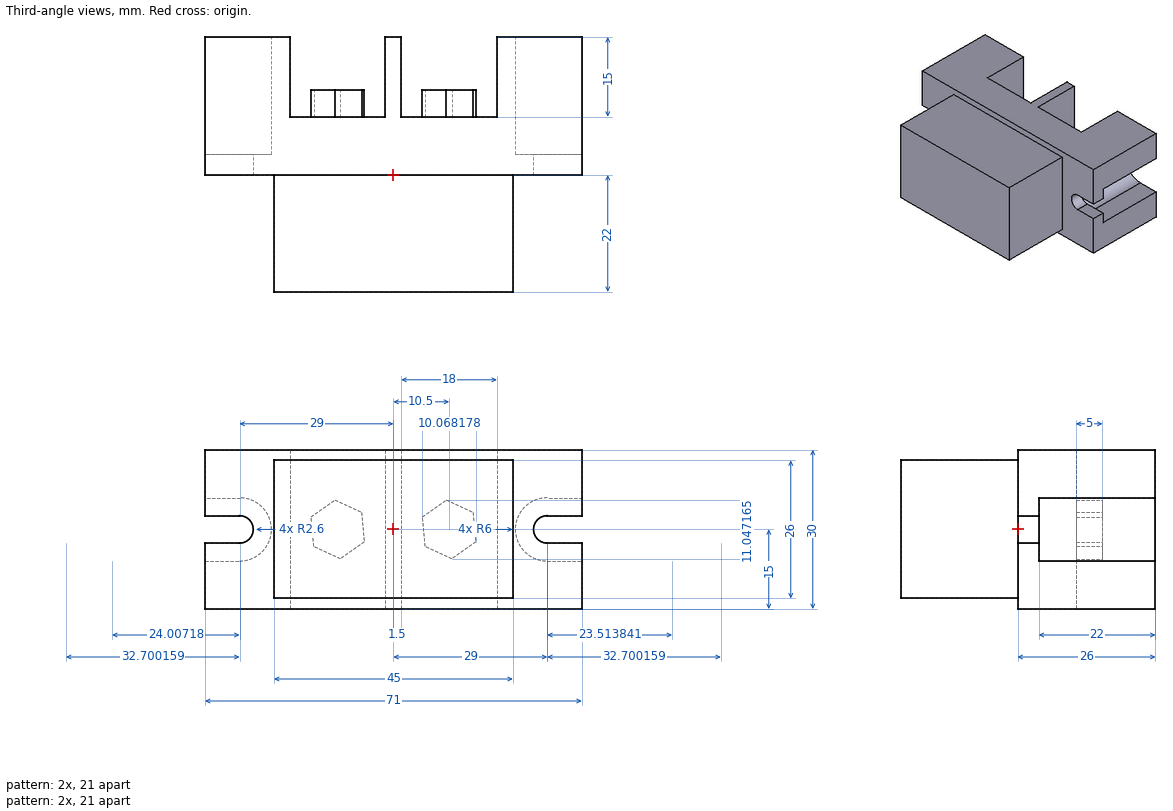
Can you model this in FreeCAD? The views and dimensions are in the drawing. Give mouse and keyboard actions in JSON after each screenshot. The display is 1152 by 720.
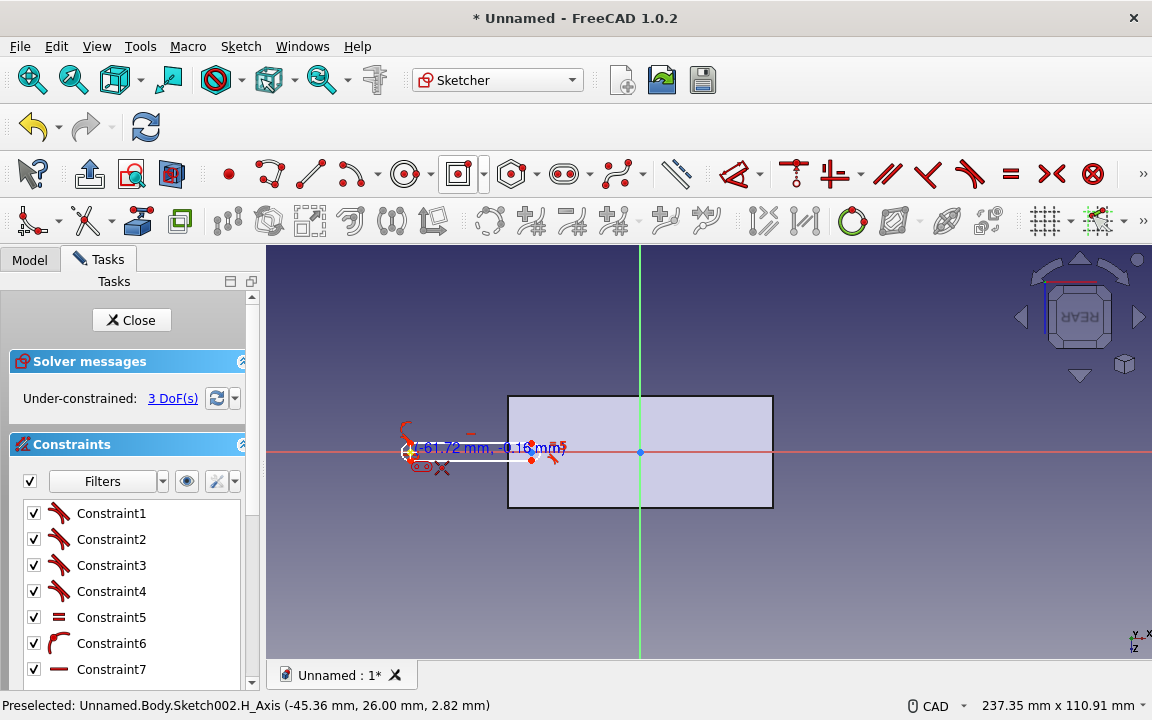
{"action": "scroll", "coordinate": [749, 452], "scroll_direction": "up", "scroll_amount": 5}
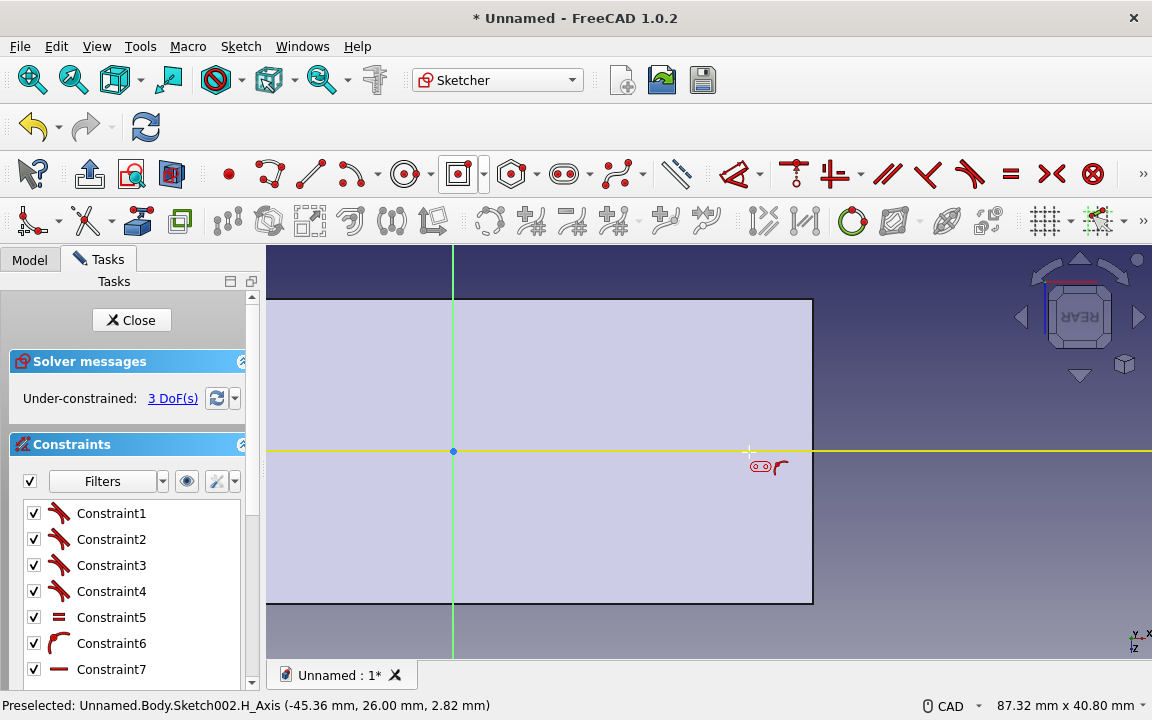
{"action": "left_click", "coordinate": [747, 451]}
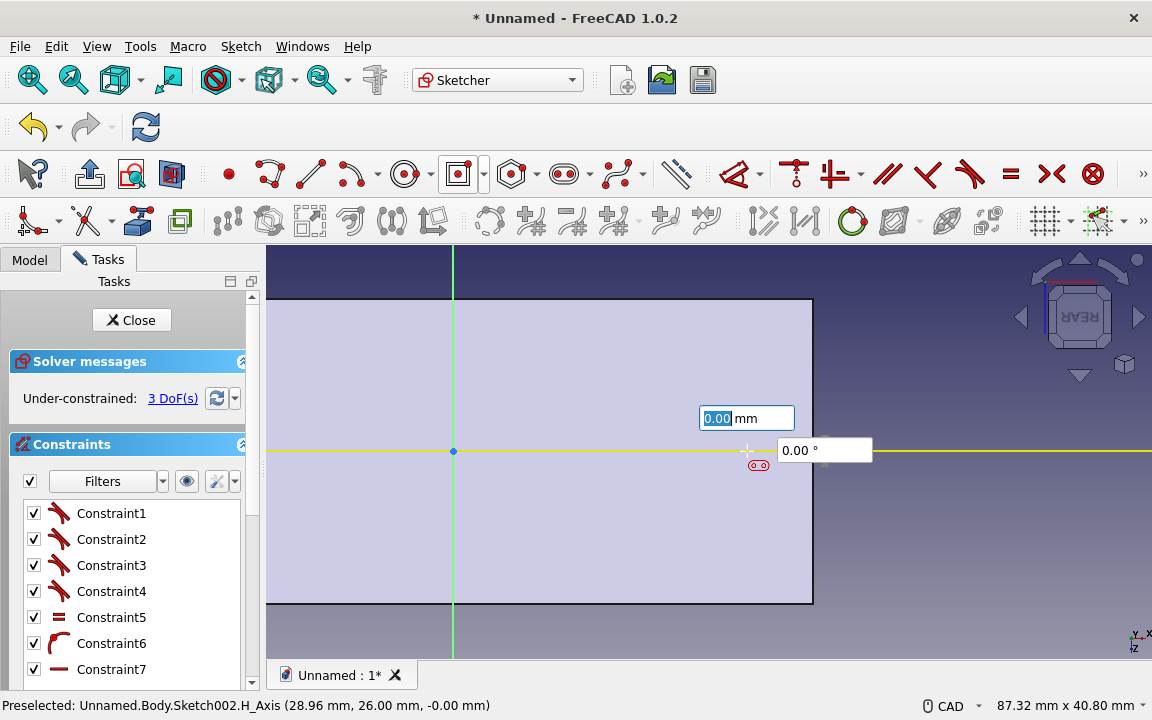
{"action": "scroll", "coordinate": [750, 452], "scroll_direction": "down", "scroll_amount": 5}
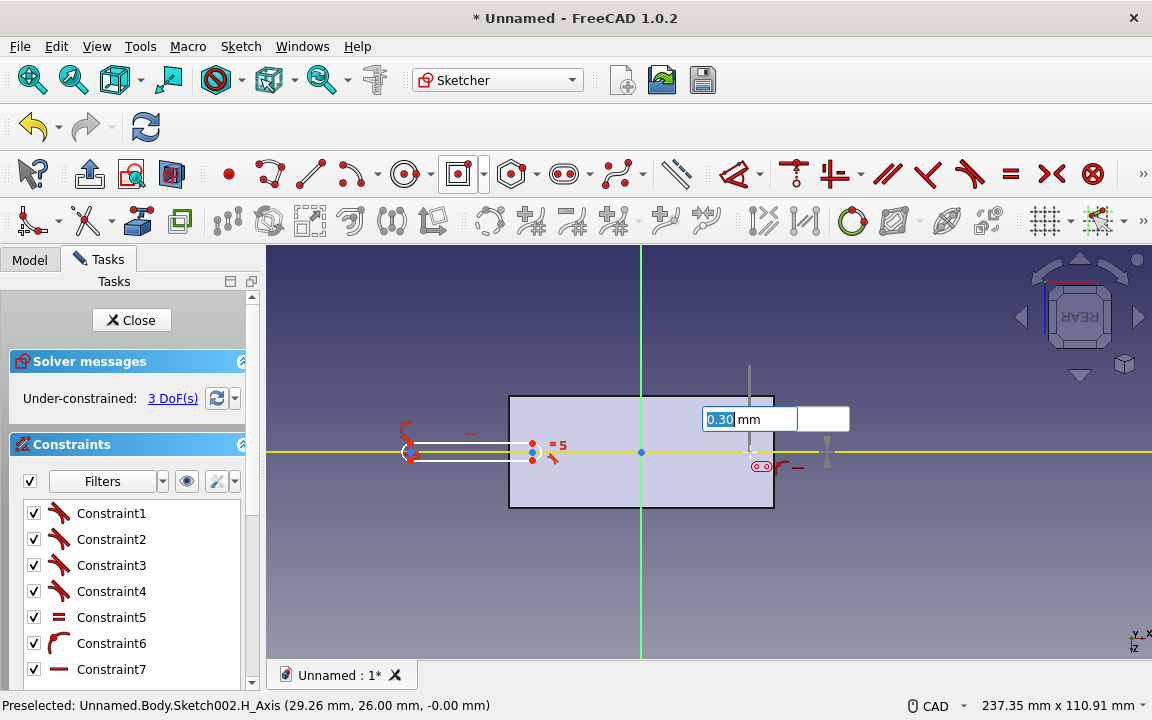
{"action": "left_click", "coordinate": [871, 443]}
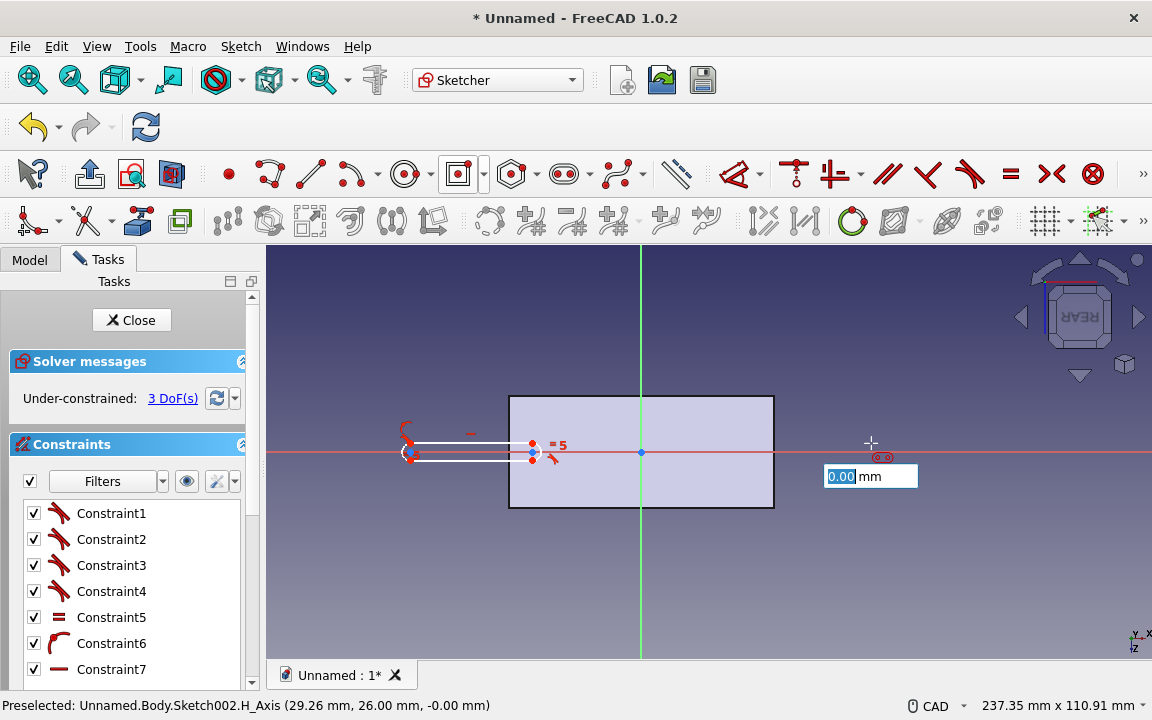
{"action": "scroll", "coordinate": [810, 442], "scroll_direction": "up", "scroll_amount": 3}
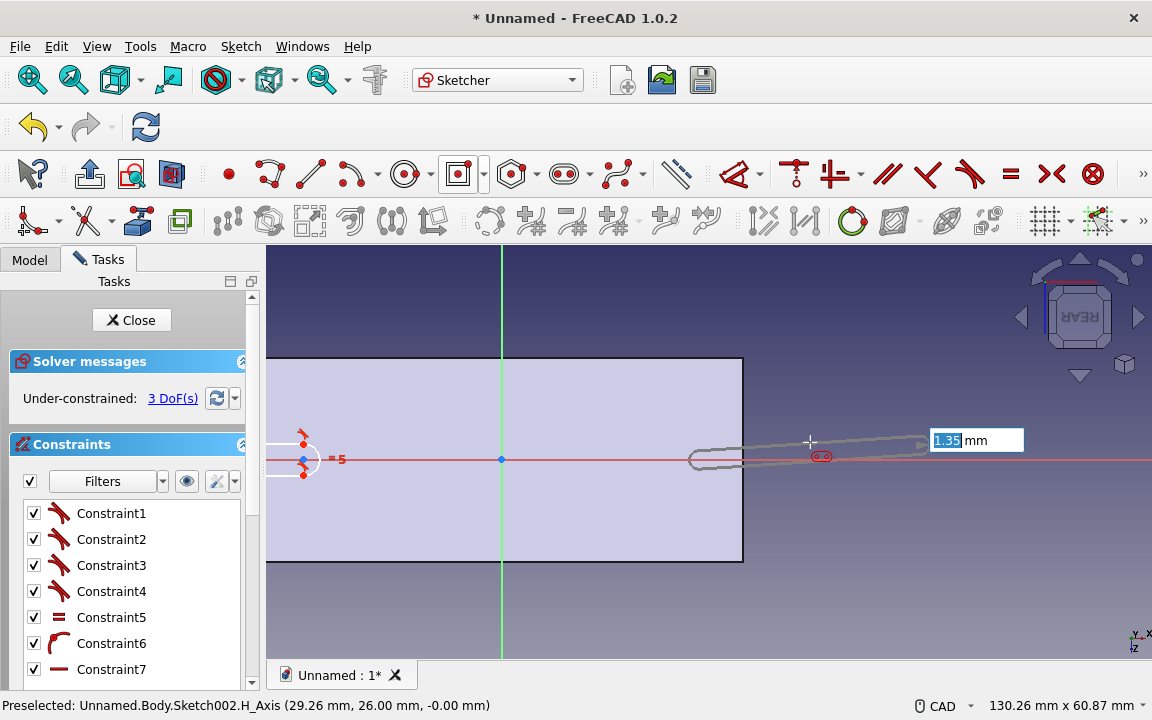
{"action": "left_click", "coordinate": [810, 442]}
{"action": "key", "text": "Escape"}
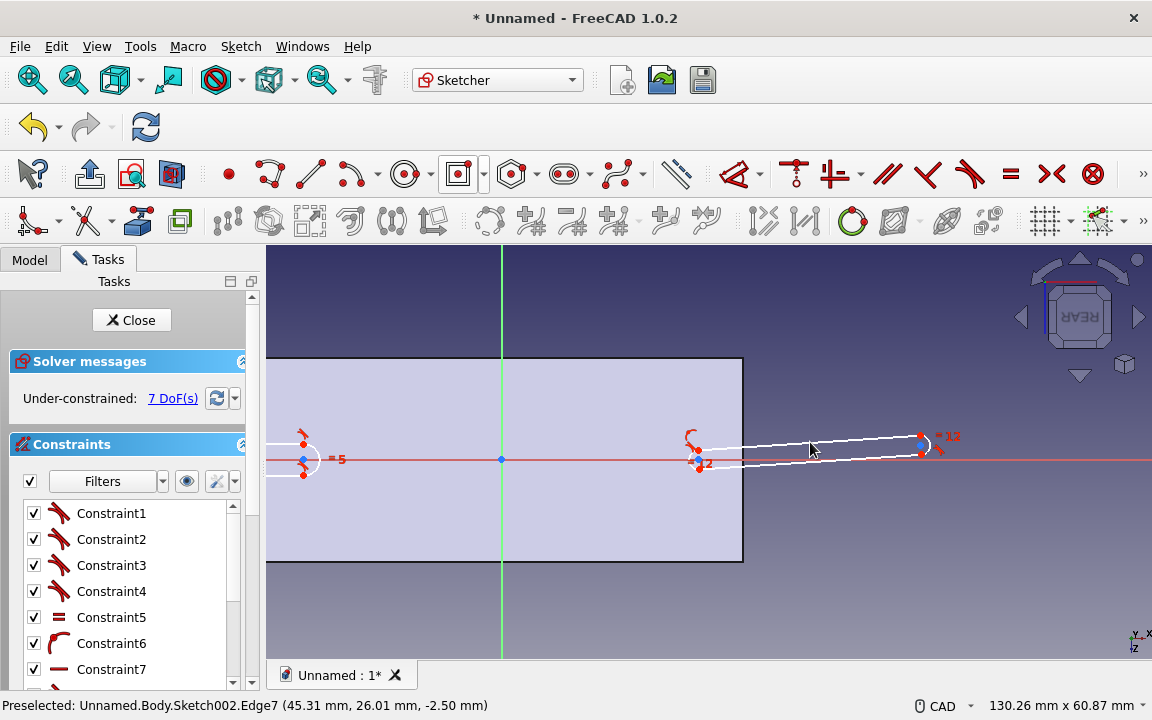
{"action": "left_click", "coordinate": [765, 446]}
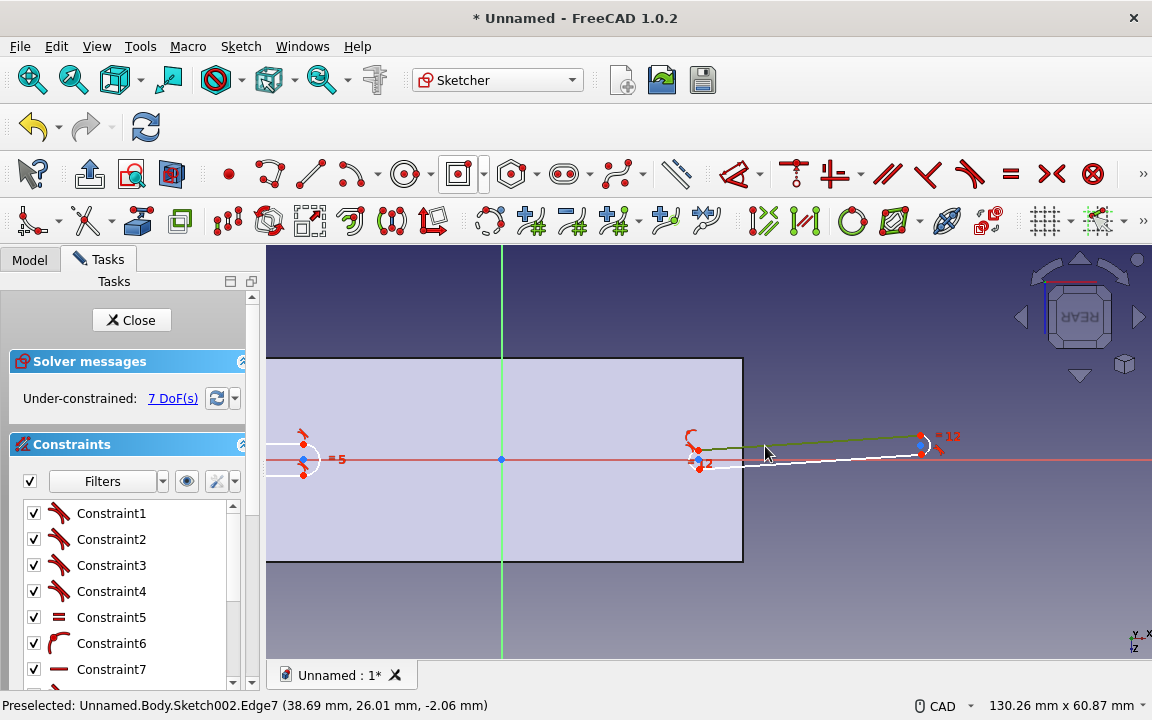
{"action": "key", "text": "h"}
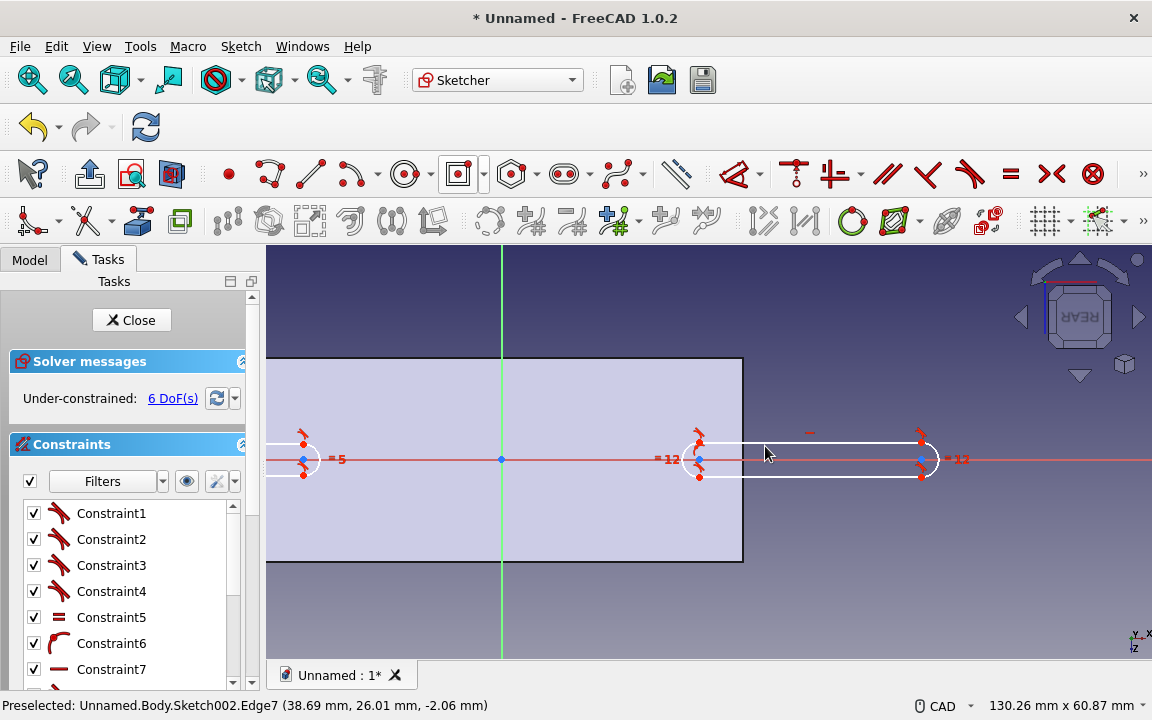
{"action": "scroll", "coordinate": [809, 442], "scroll_direction": "down", "scroll_amount": 3}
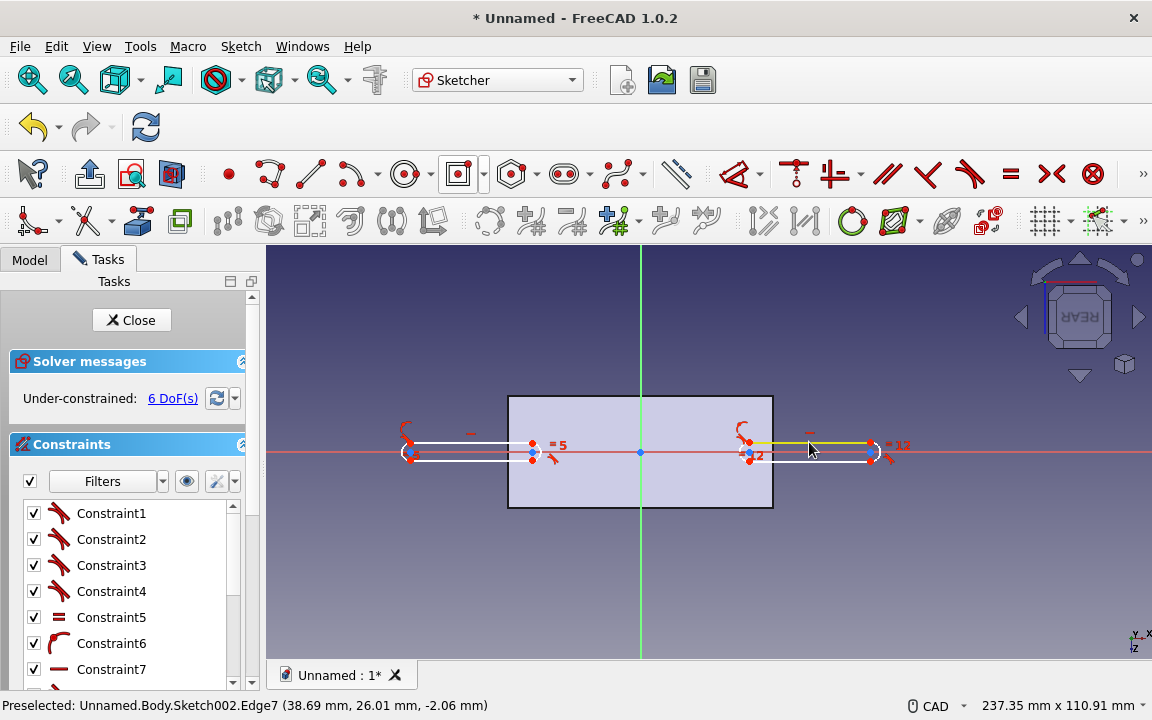
{"action": "scroll", "coordinate": [403, 447], "scroll_direction": "up", "scroll_amount": 6}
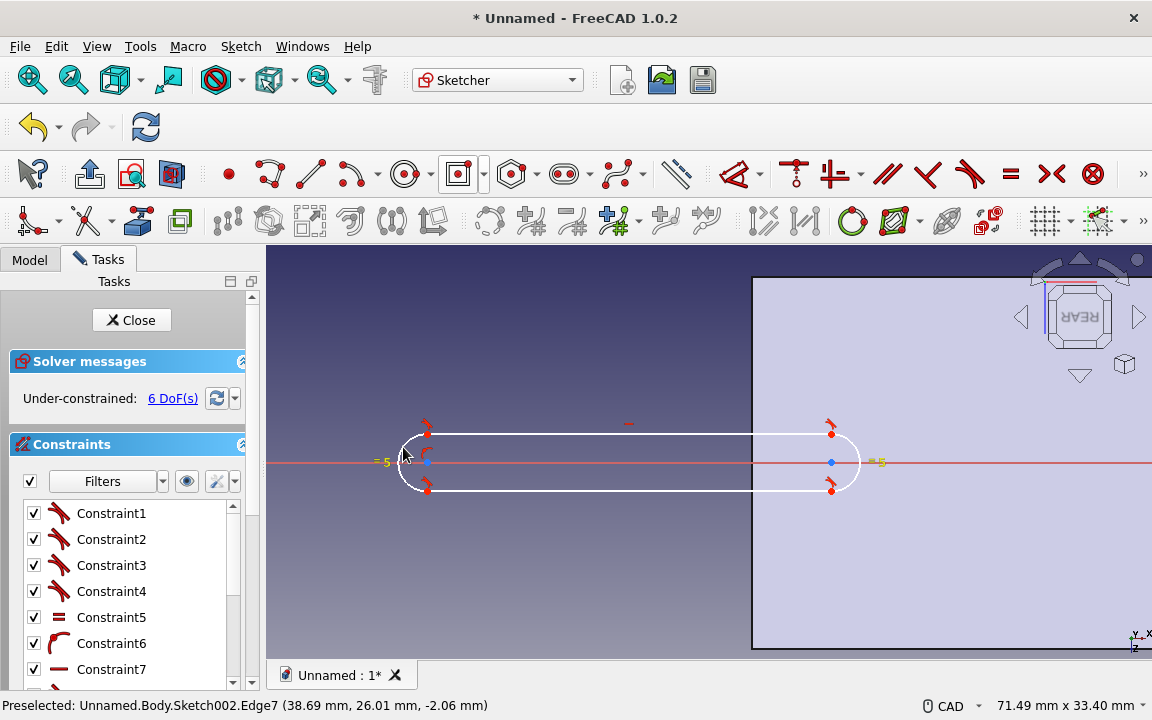
{"action": "left_click", "coordinate": [404, 446]}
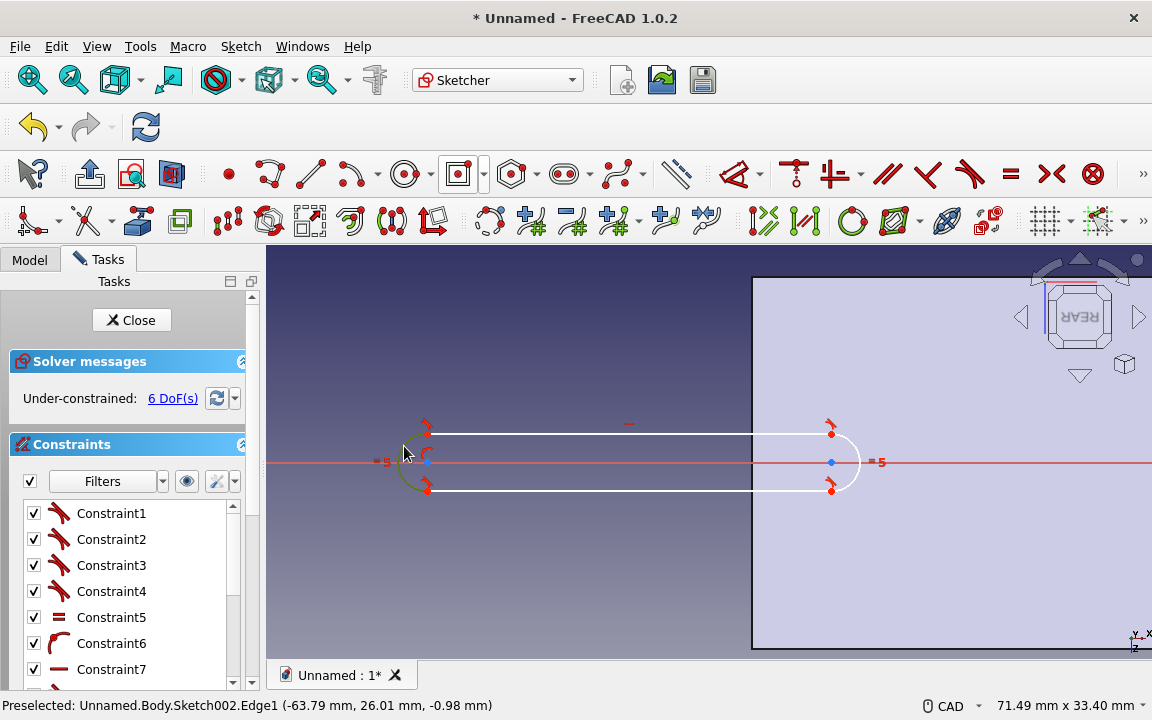
{"action": "scroll", "coordinate": [403, 447], "scroll_direction": "down", "scroll_amount": 6}